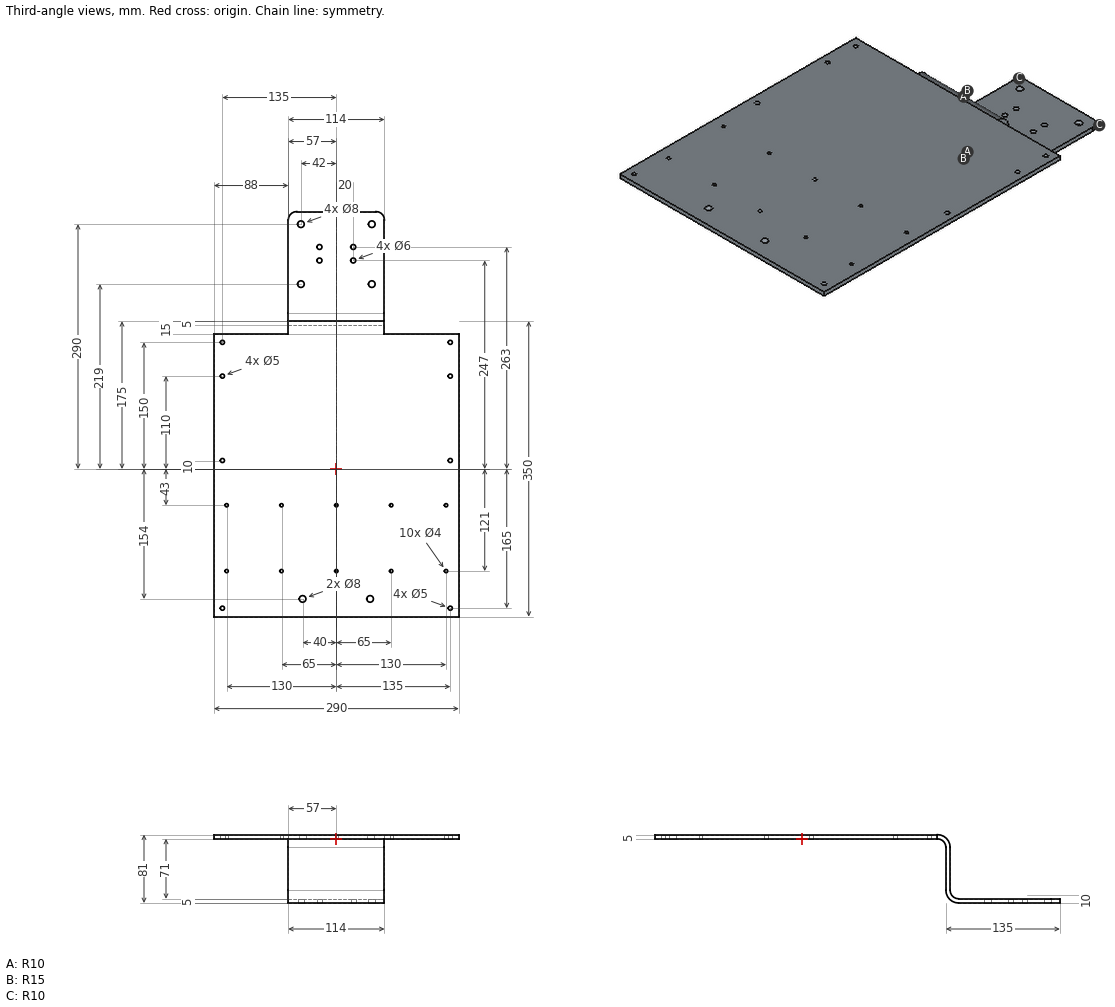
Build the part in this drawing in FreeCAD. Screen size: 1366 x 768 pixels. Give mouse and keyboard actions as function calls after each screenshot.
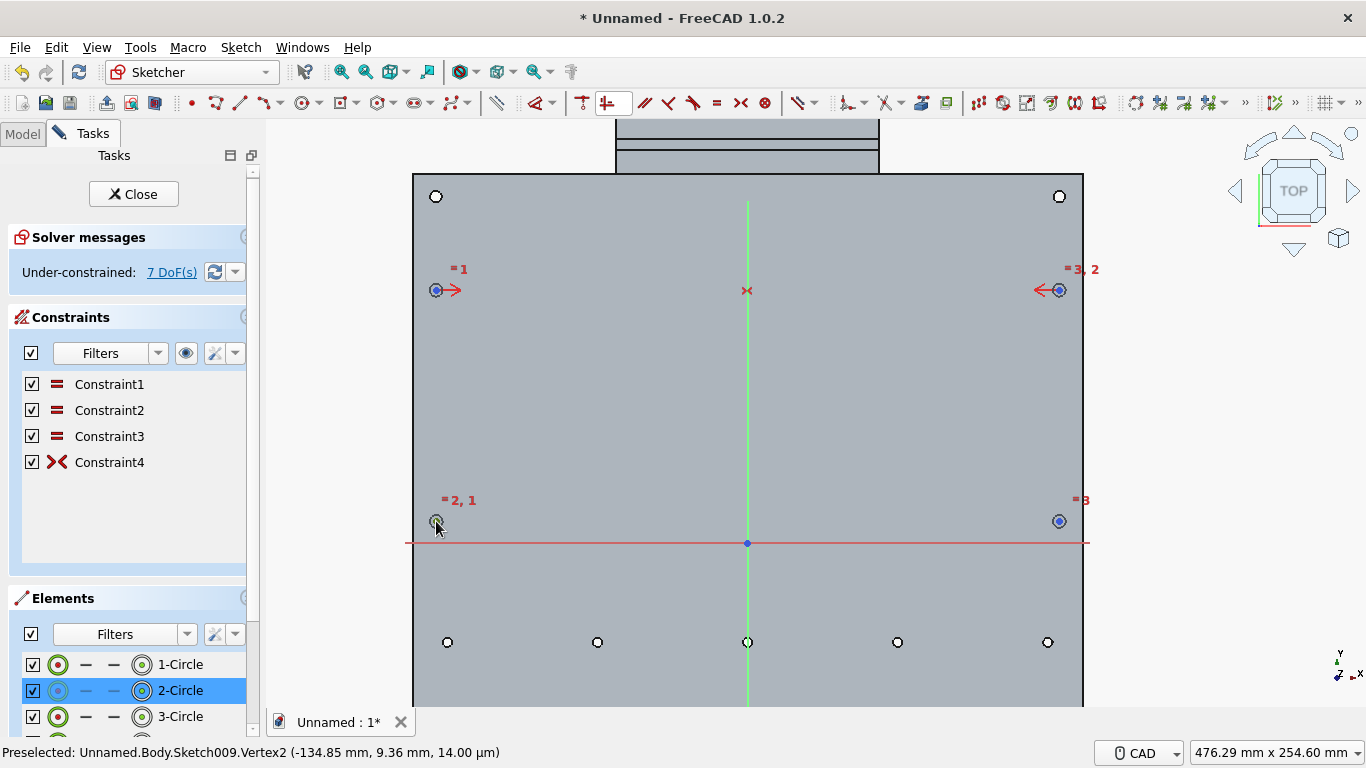
click(1059, 521)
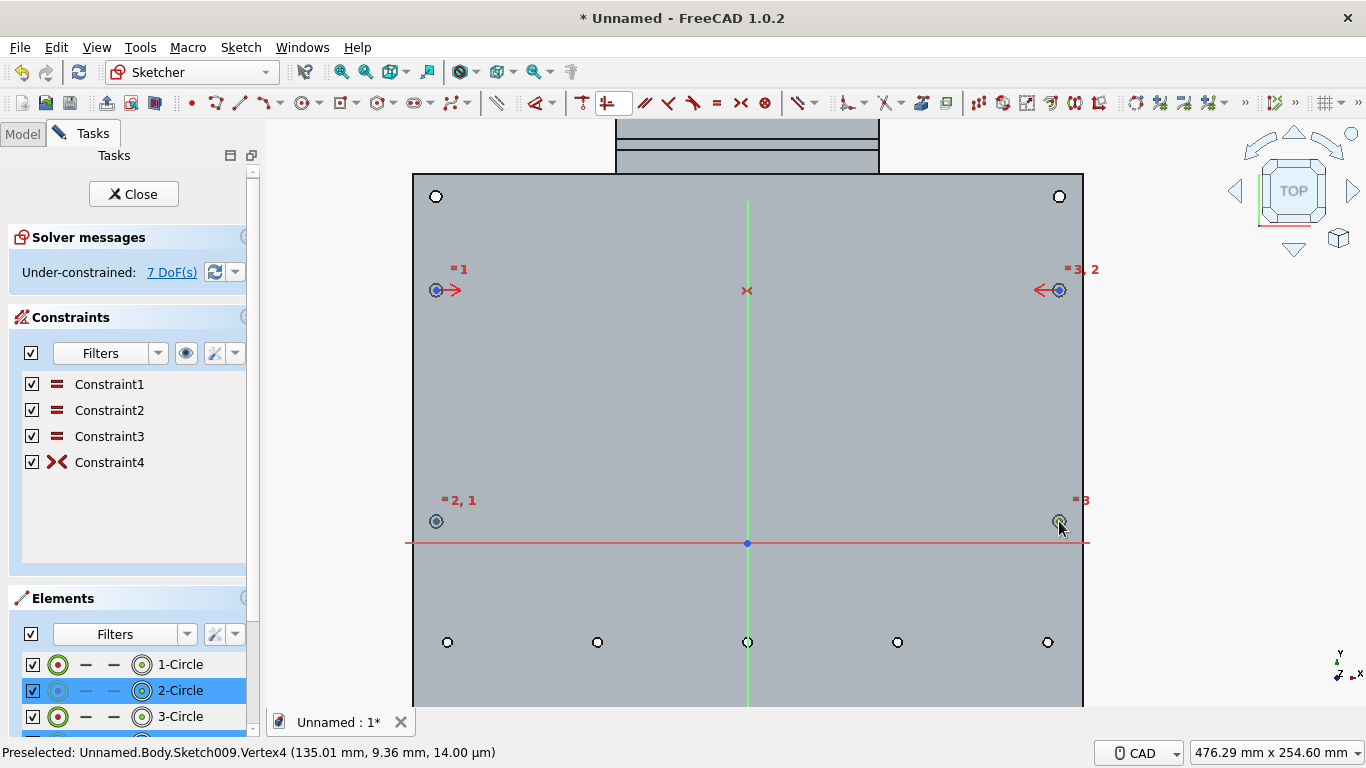
click(748, 641)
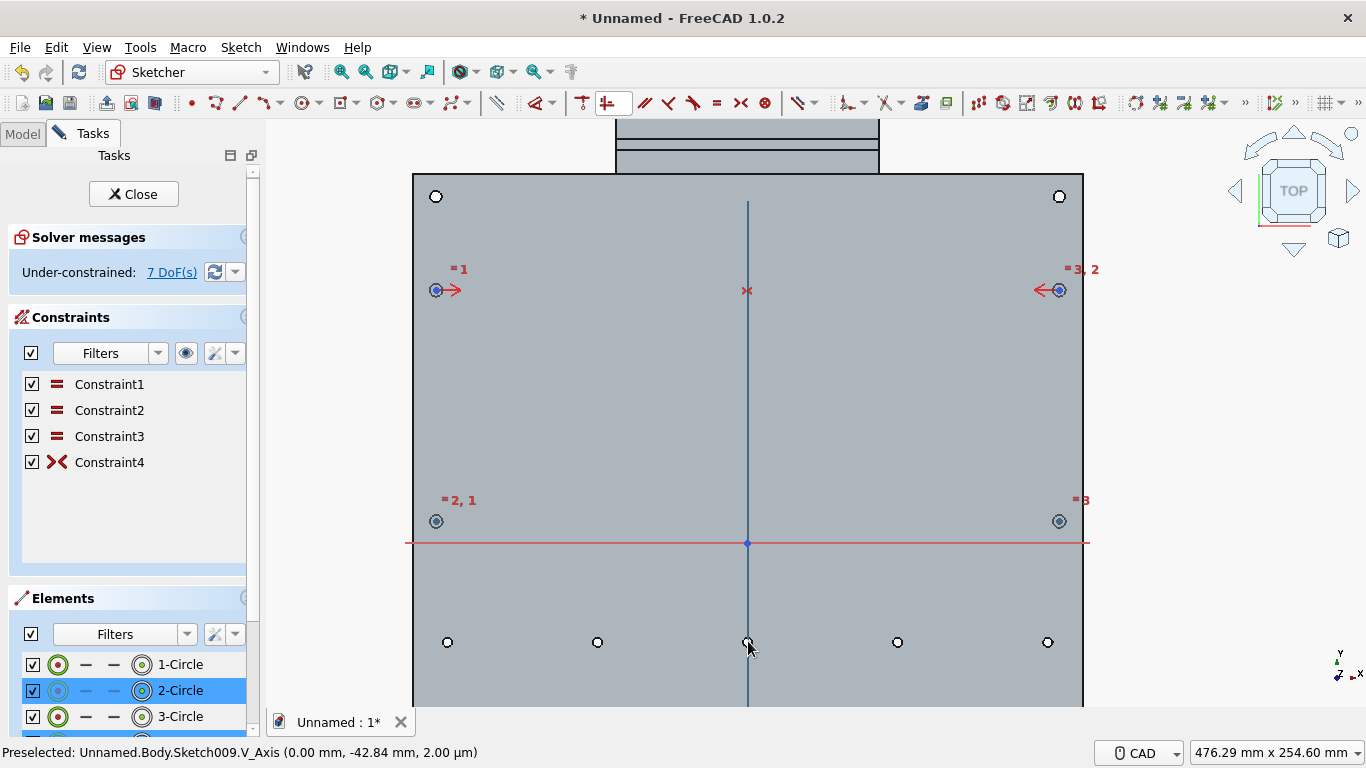
key(s)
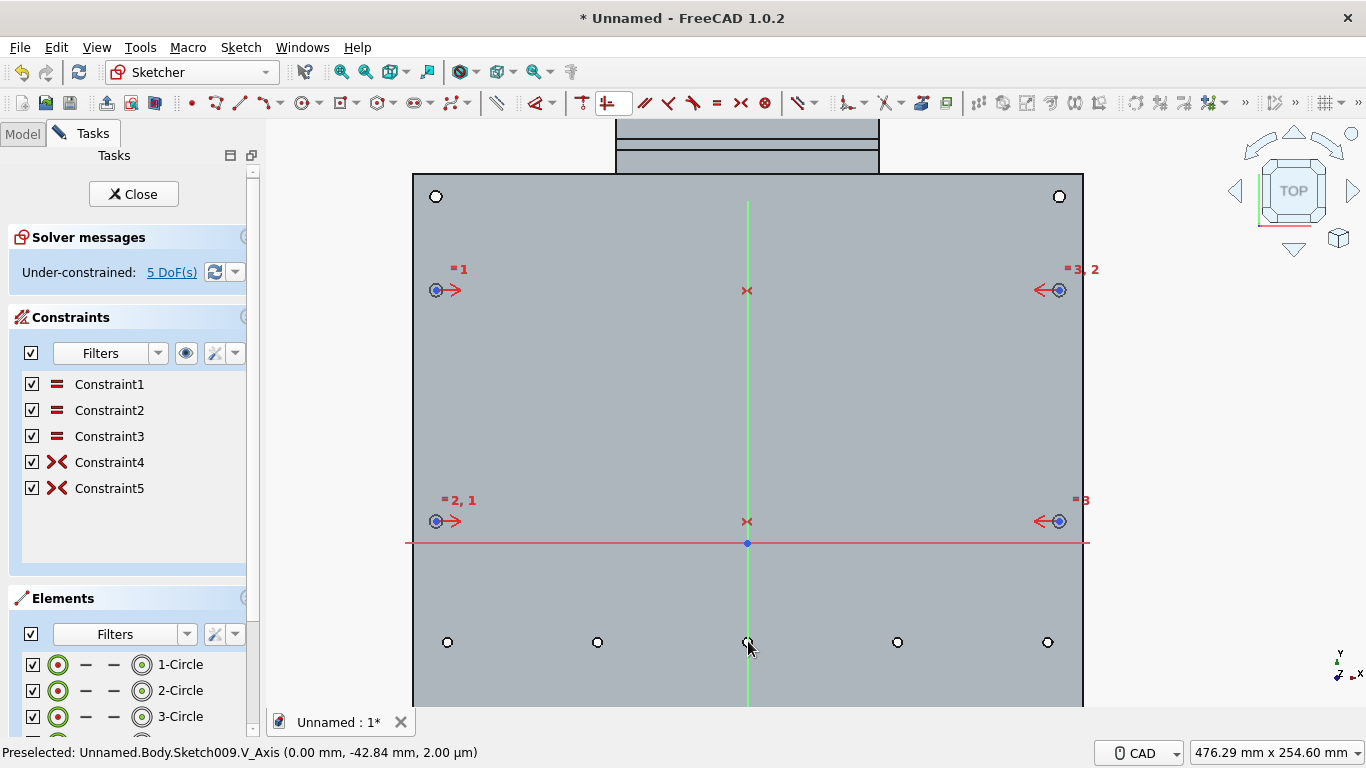
click(536, 104)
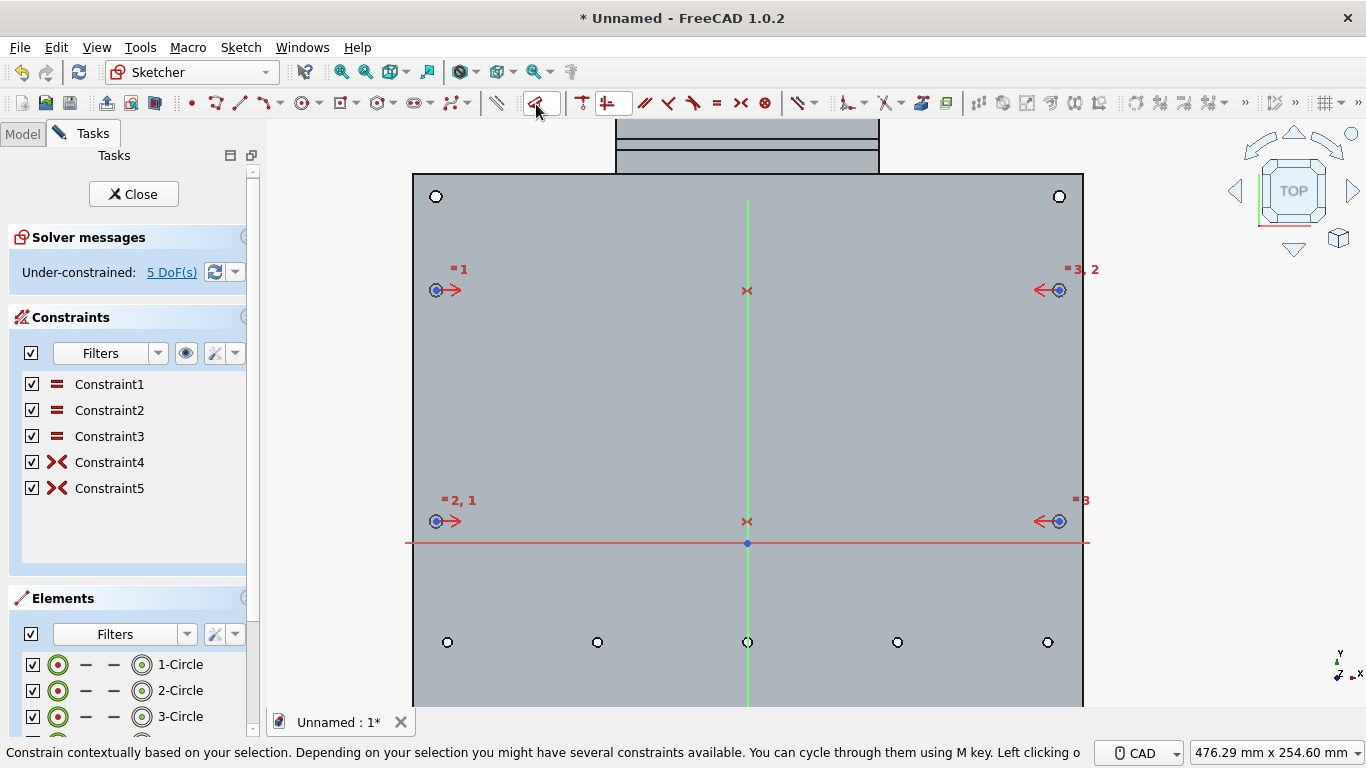
scroll(432, 286, up, 7)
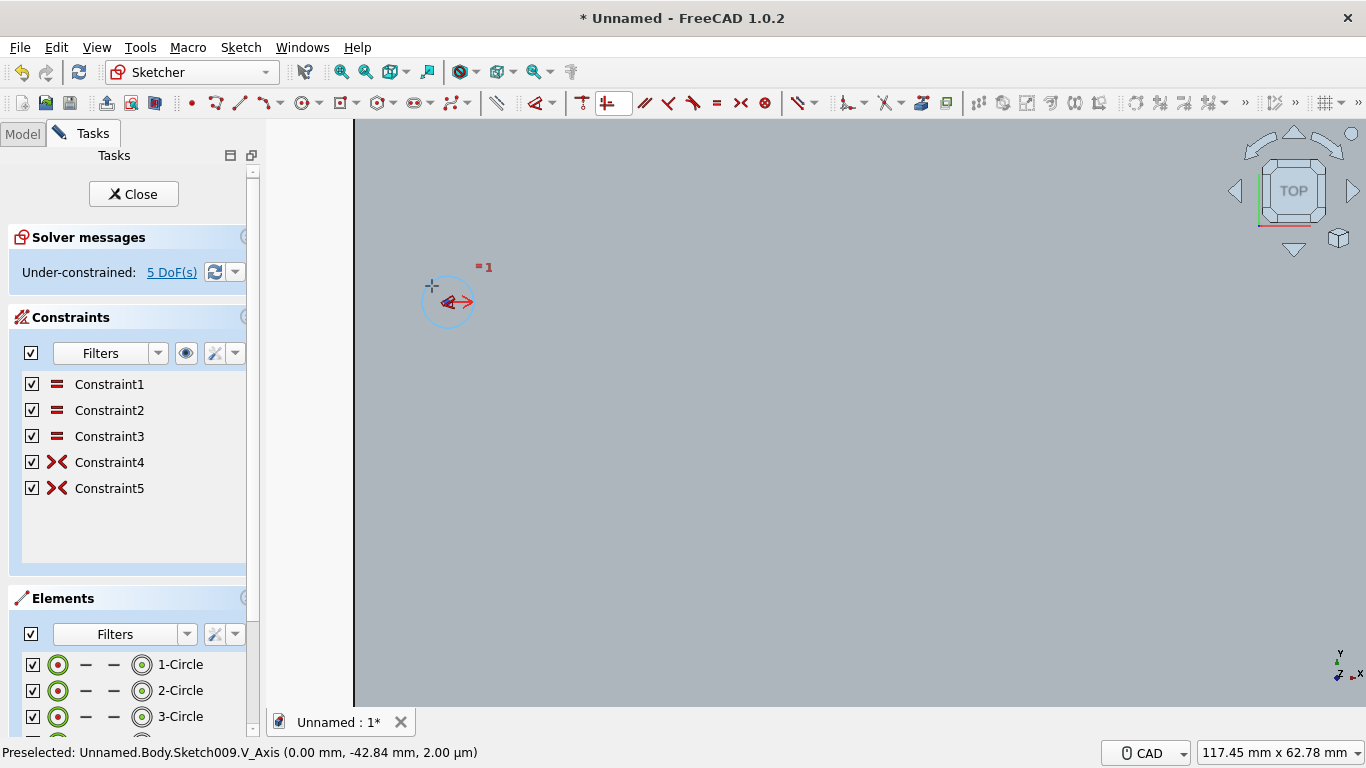
click(430, 284)
click(408, 261)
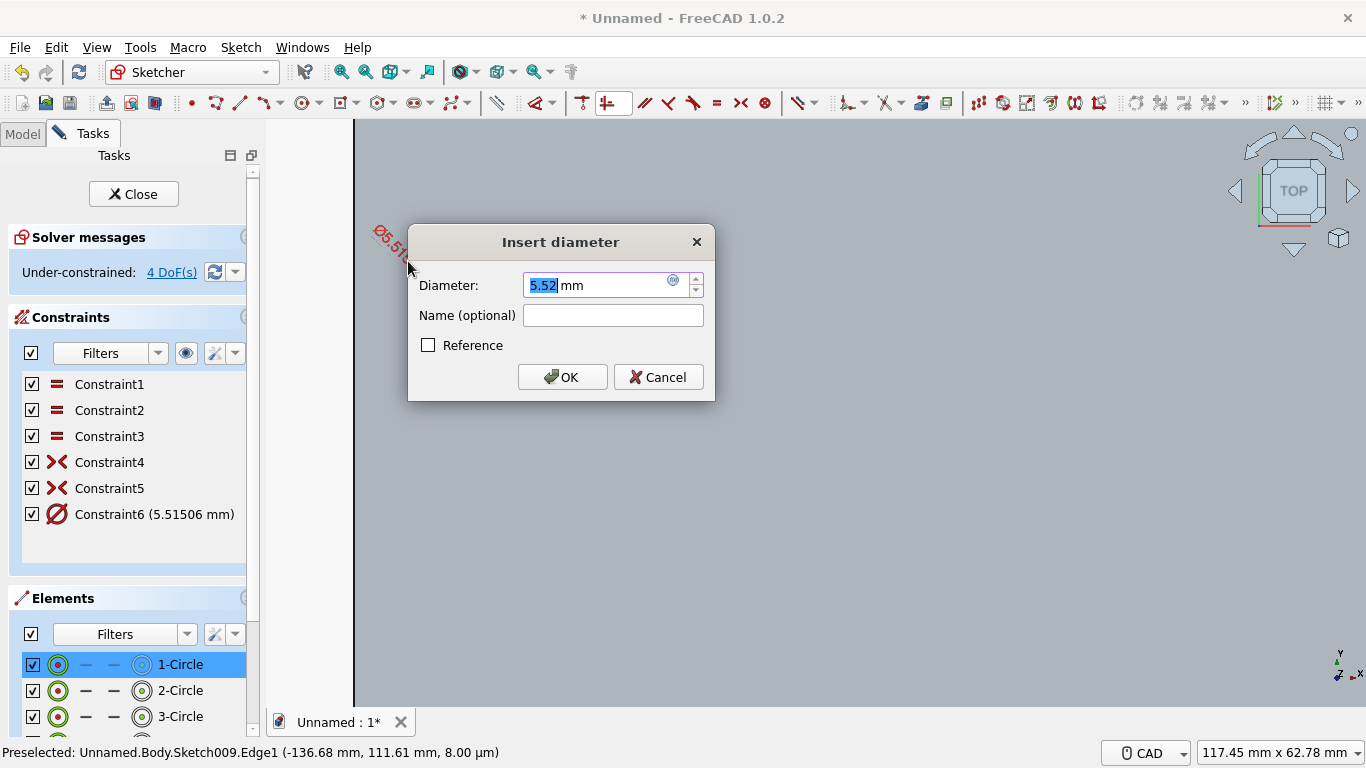
text(5)
key(Return)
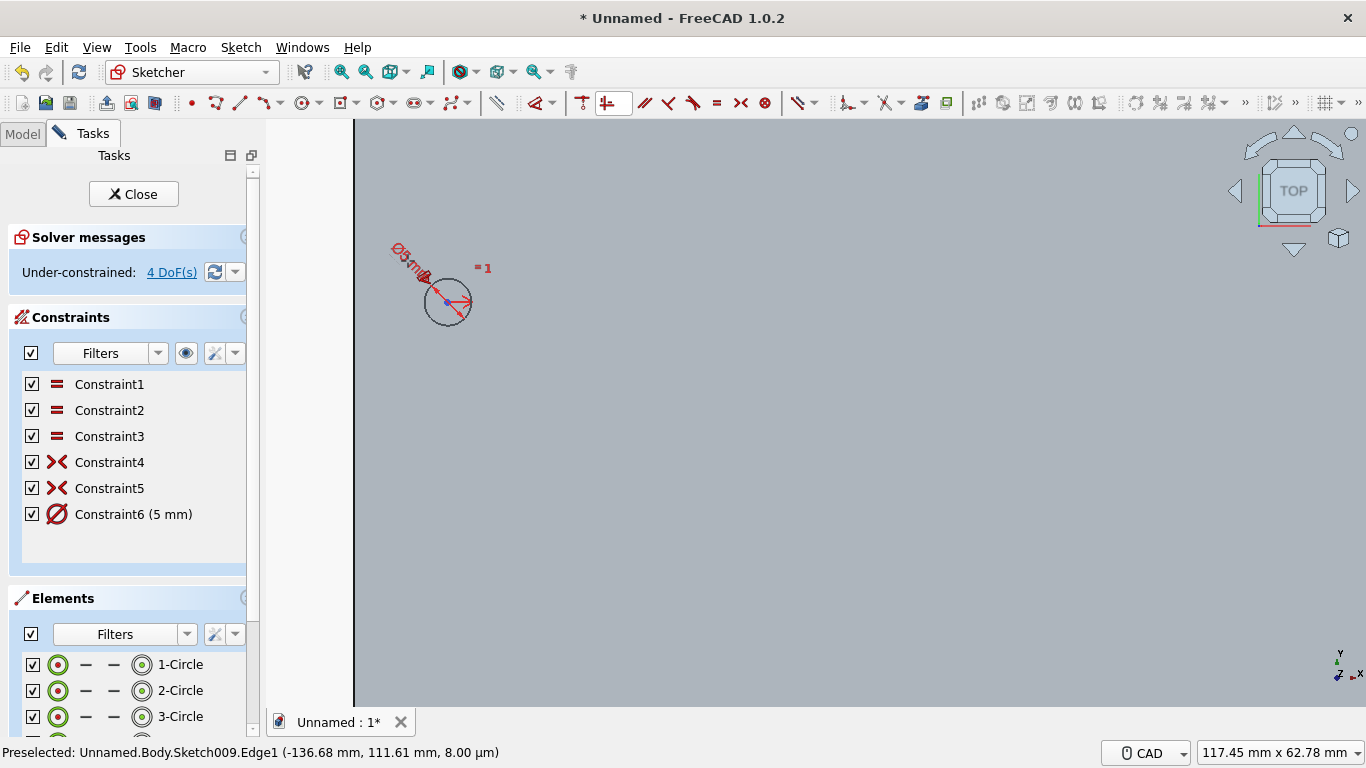
scroll(432, 286, down, 7)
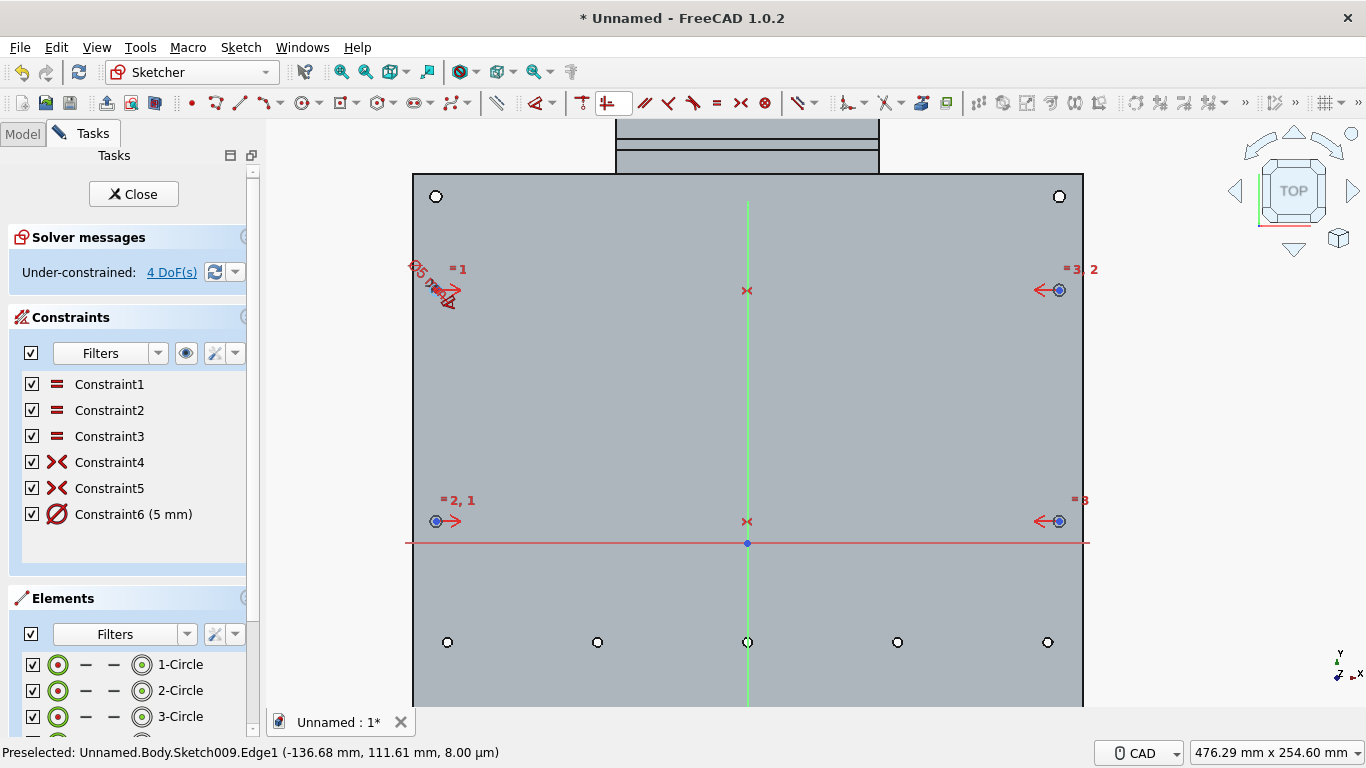
scroll(436, 521, up, 3)